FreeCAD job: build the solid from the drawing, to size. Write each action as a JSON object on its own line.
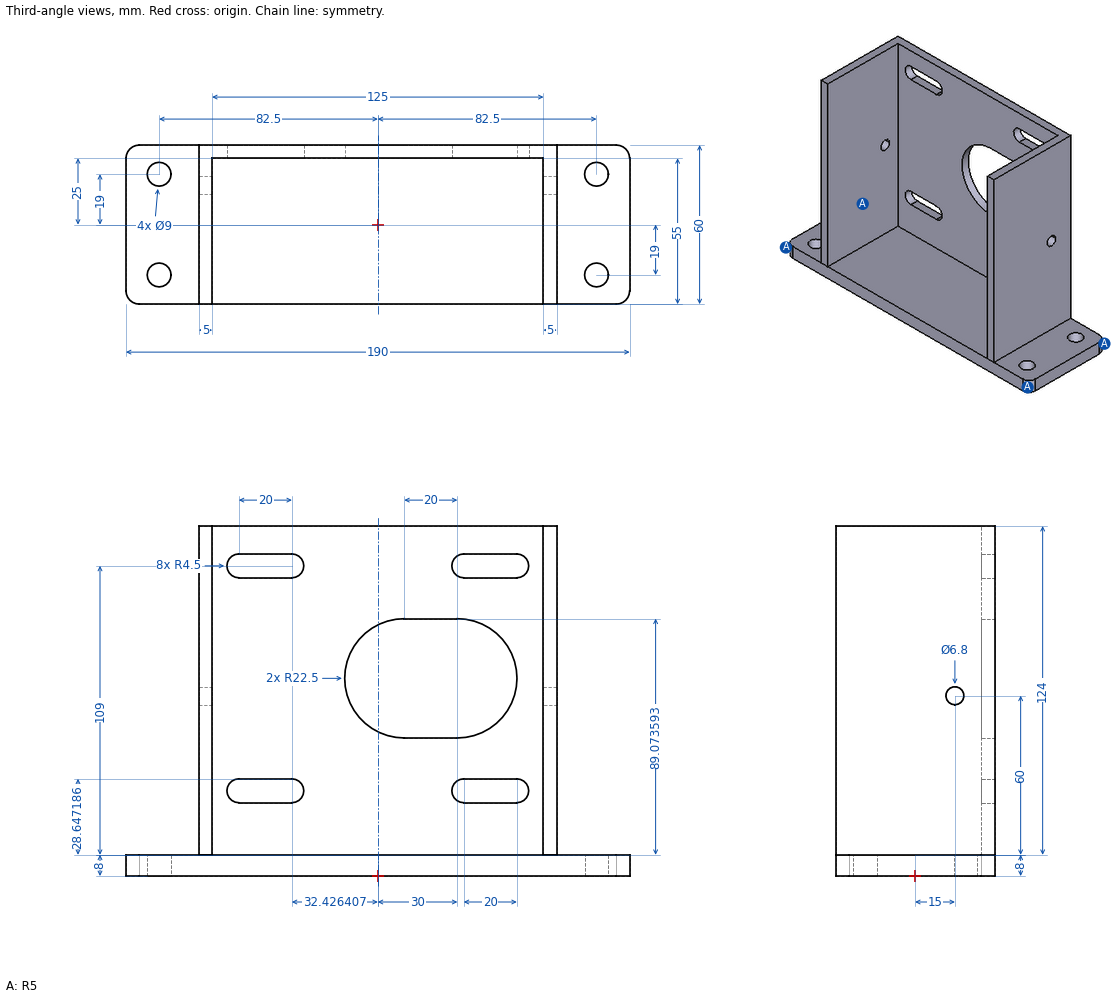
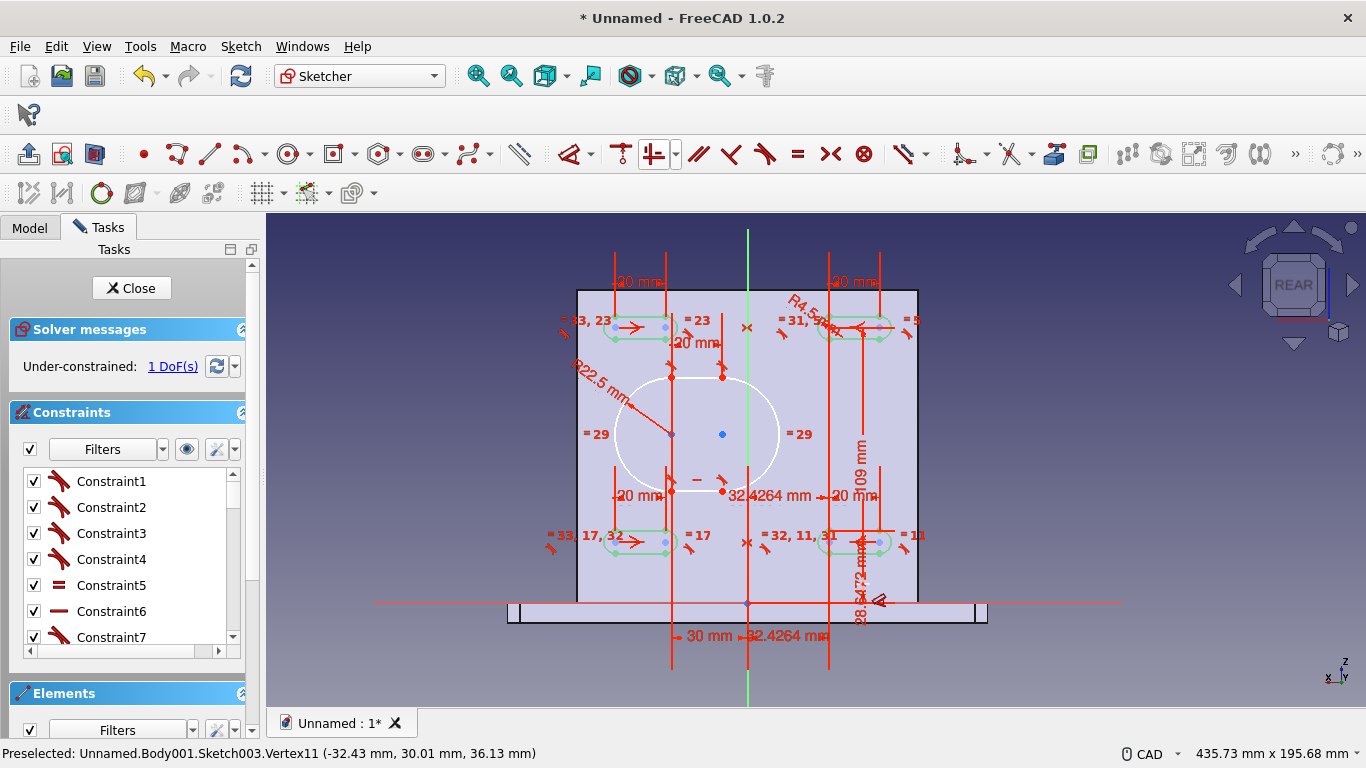
{"action": "left_click", "coordinate": [672, 378]}
{"action": "left_click", "coordinate": [638, 439]}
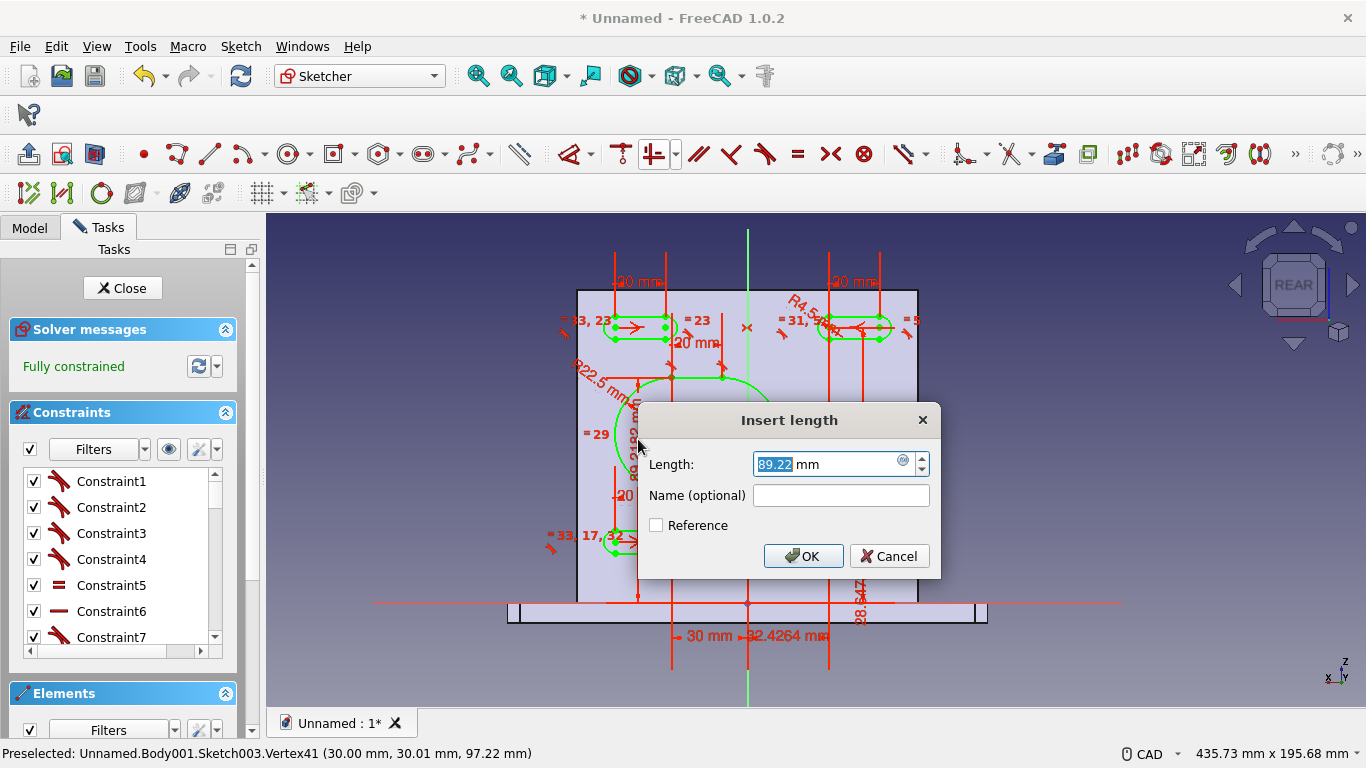
{"action": "type", "text": "89.073593"}
{"action": "key", "text": "Return"}
{"action": "key", "text": "Escape"}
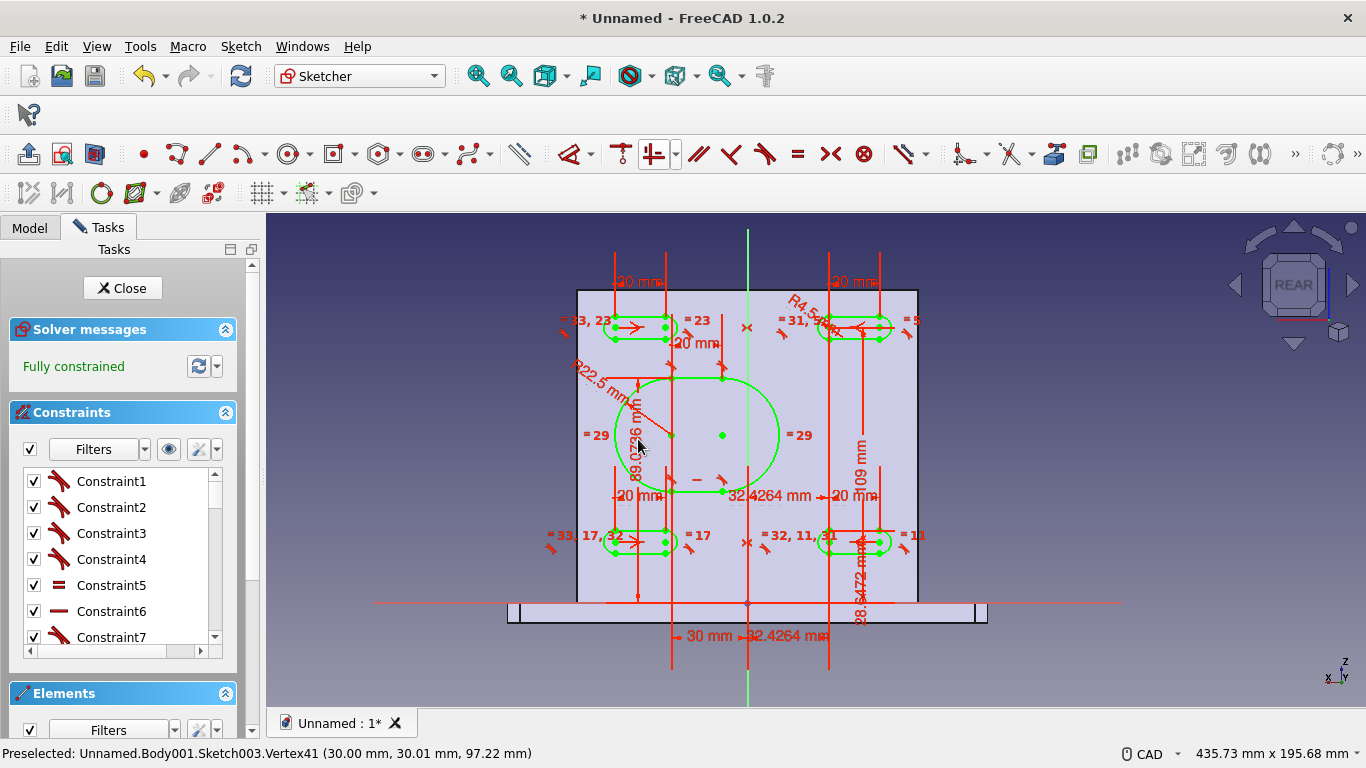
{"action": "left_click", "coordinate": [123, 288]}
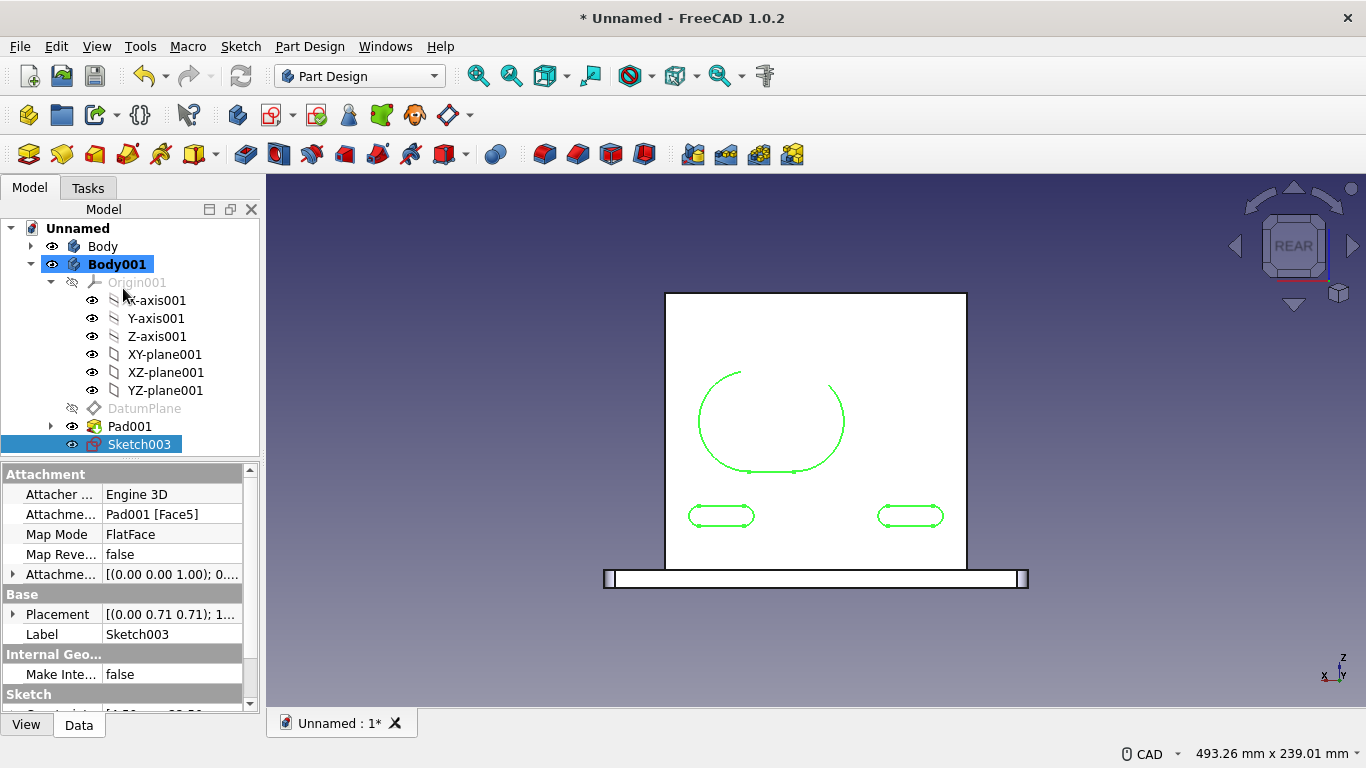
{"action": "left_click", "coordinate": [246, 154]}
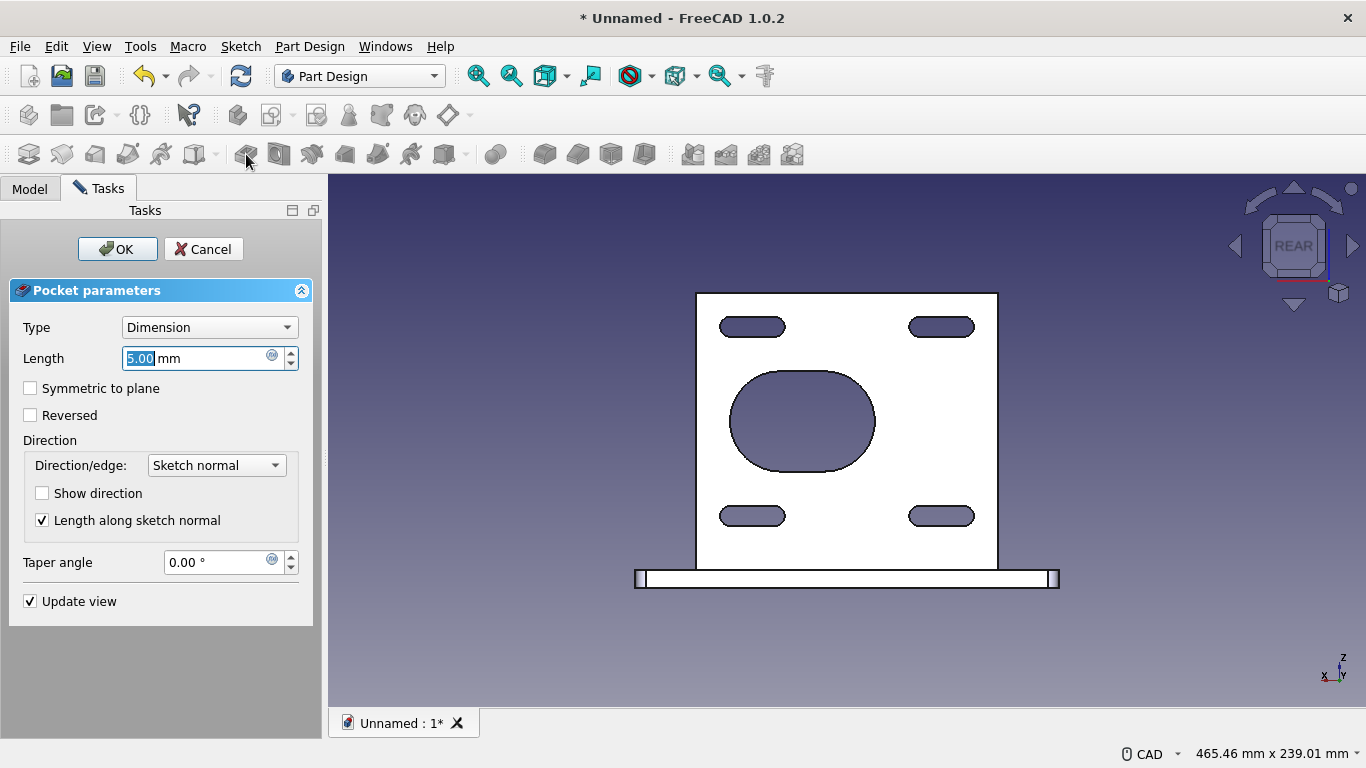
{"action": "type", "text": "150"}
{"action": "key", "text": "Tab"}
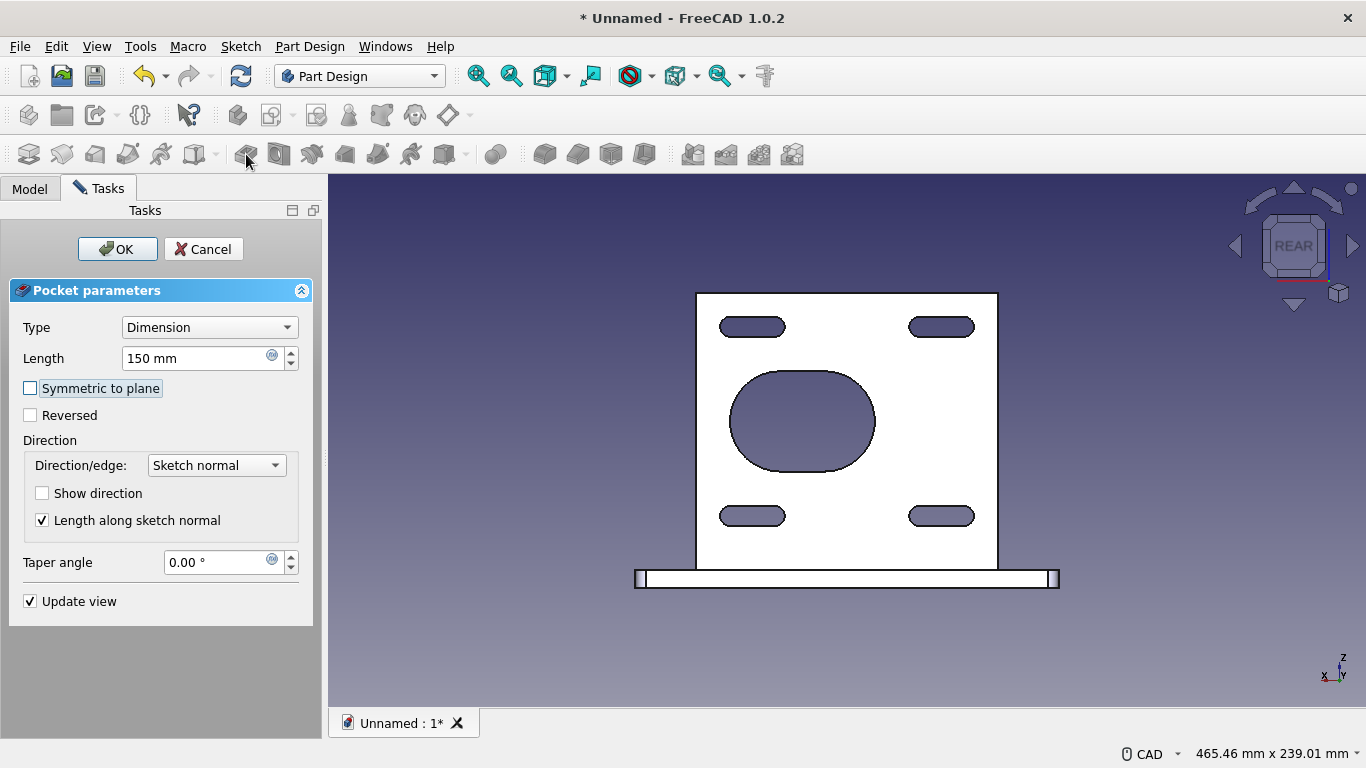
{"action": "left_click", "coordinate": [118, 249]}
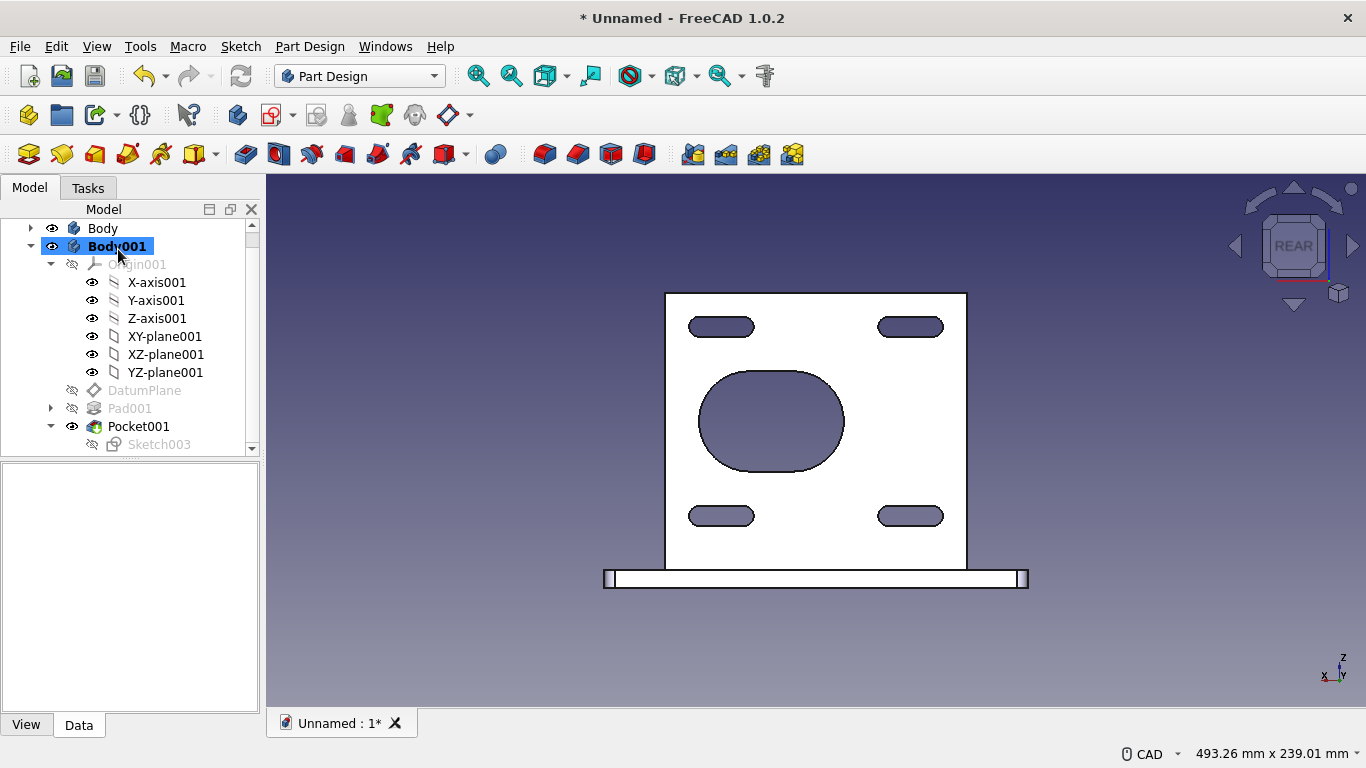
{"action": "key", "text": "0"}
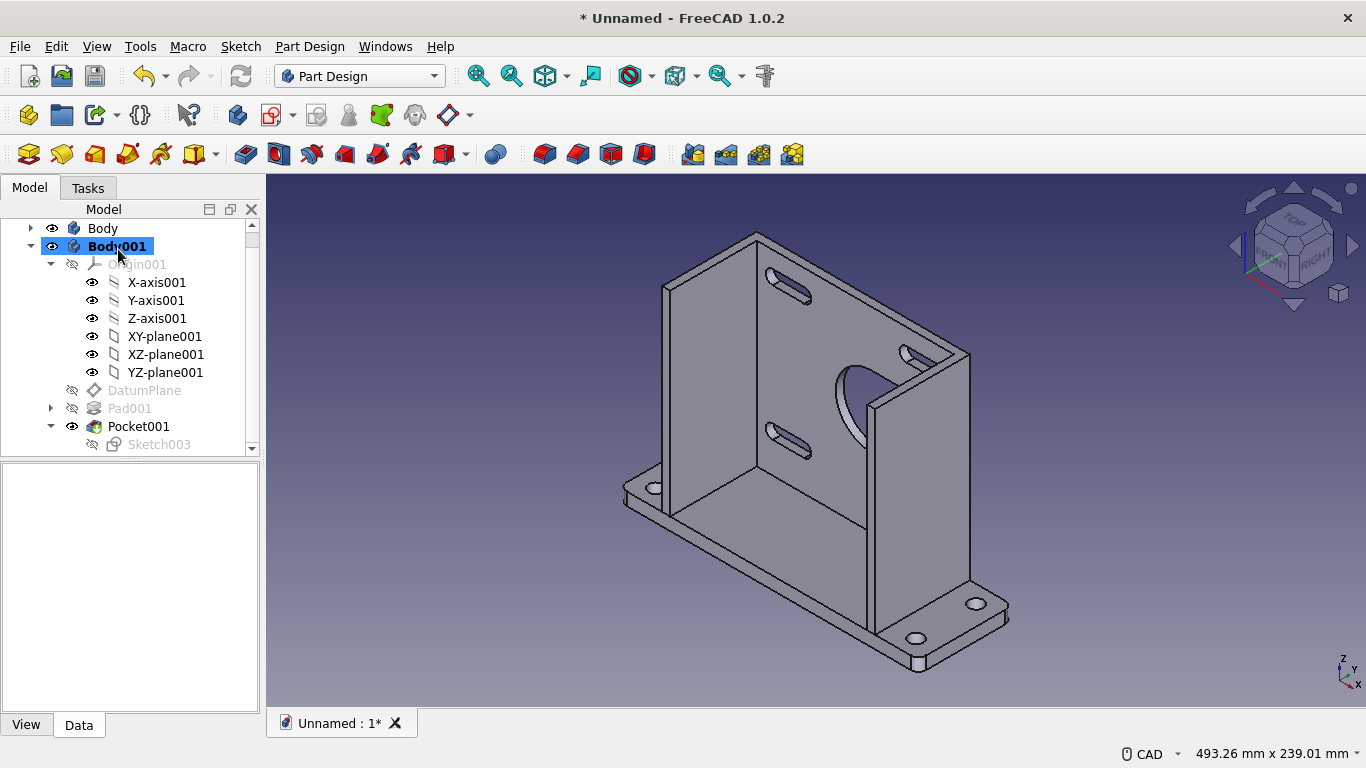
{"action": "left_click", "coordinate": [922, 461]}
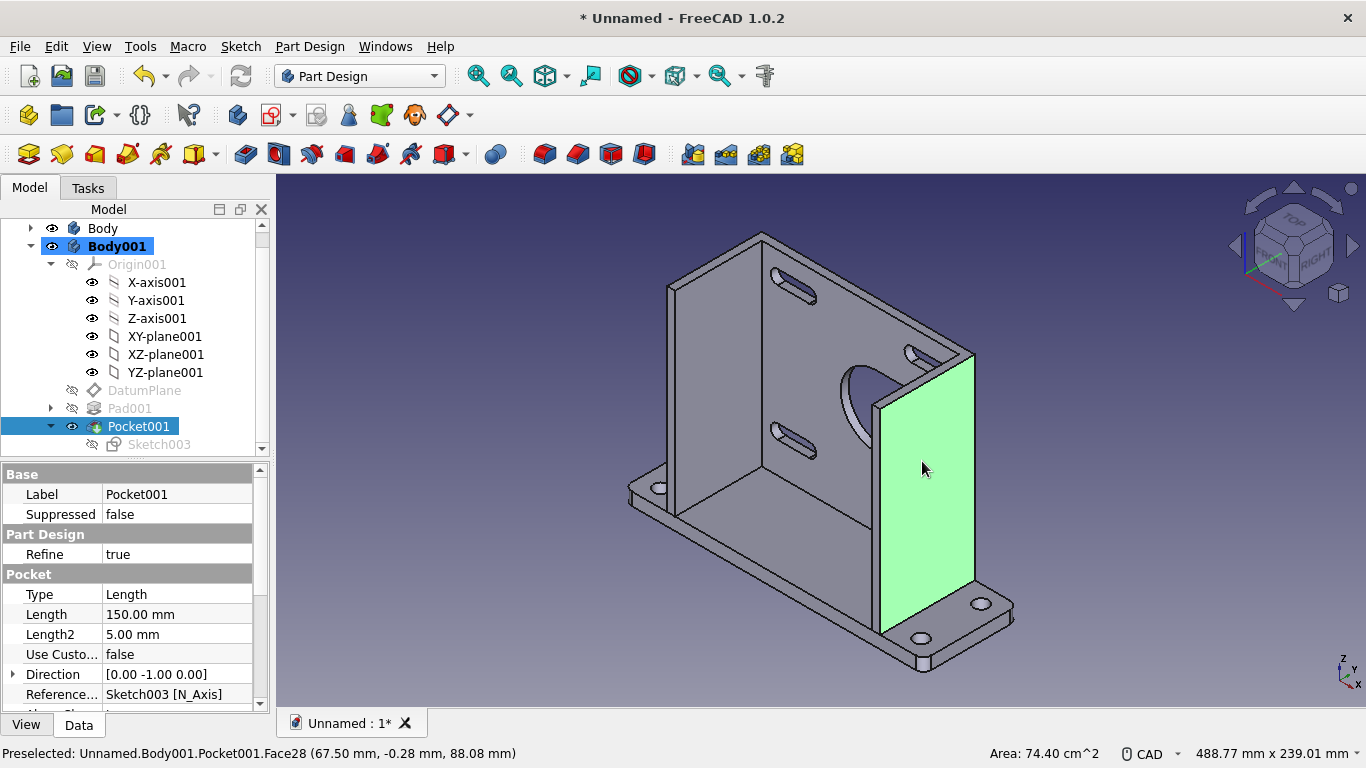
{"action": "left_click", "coordinate": [270, 116]}